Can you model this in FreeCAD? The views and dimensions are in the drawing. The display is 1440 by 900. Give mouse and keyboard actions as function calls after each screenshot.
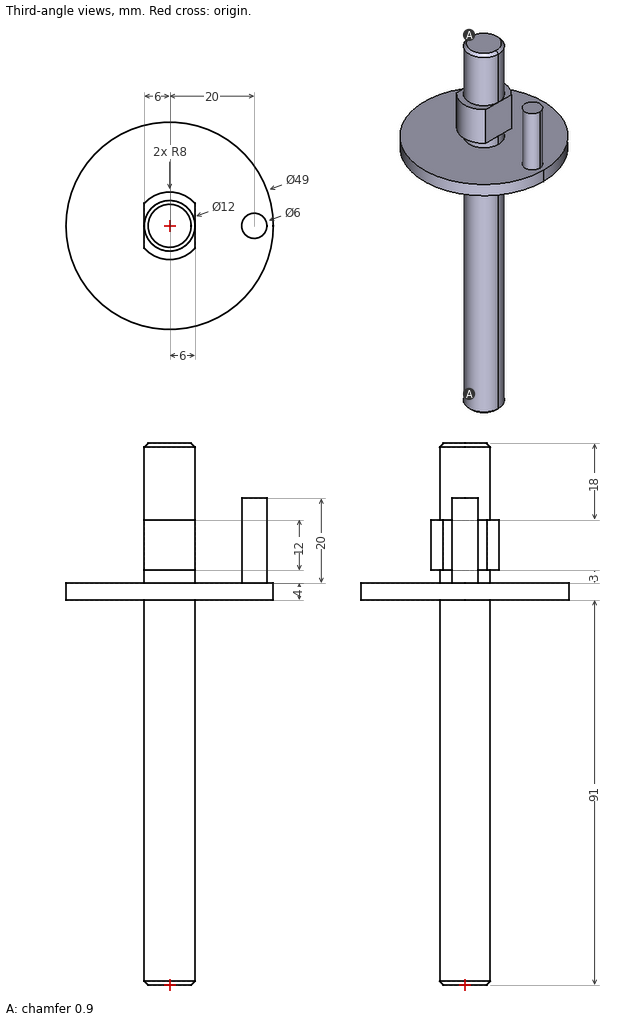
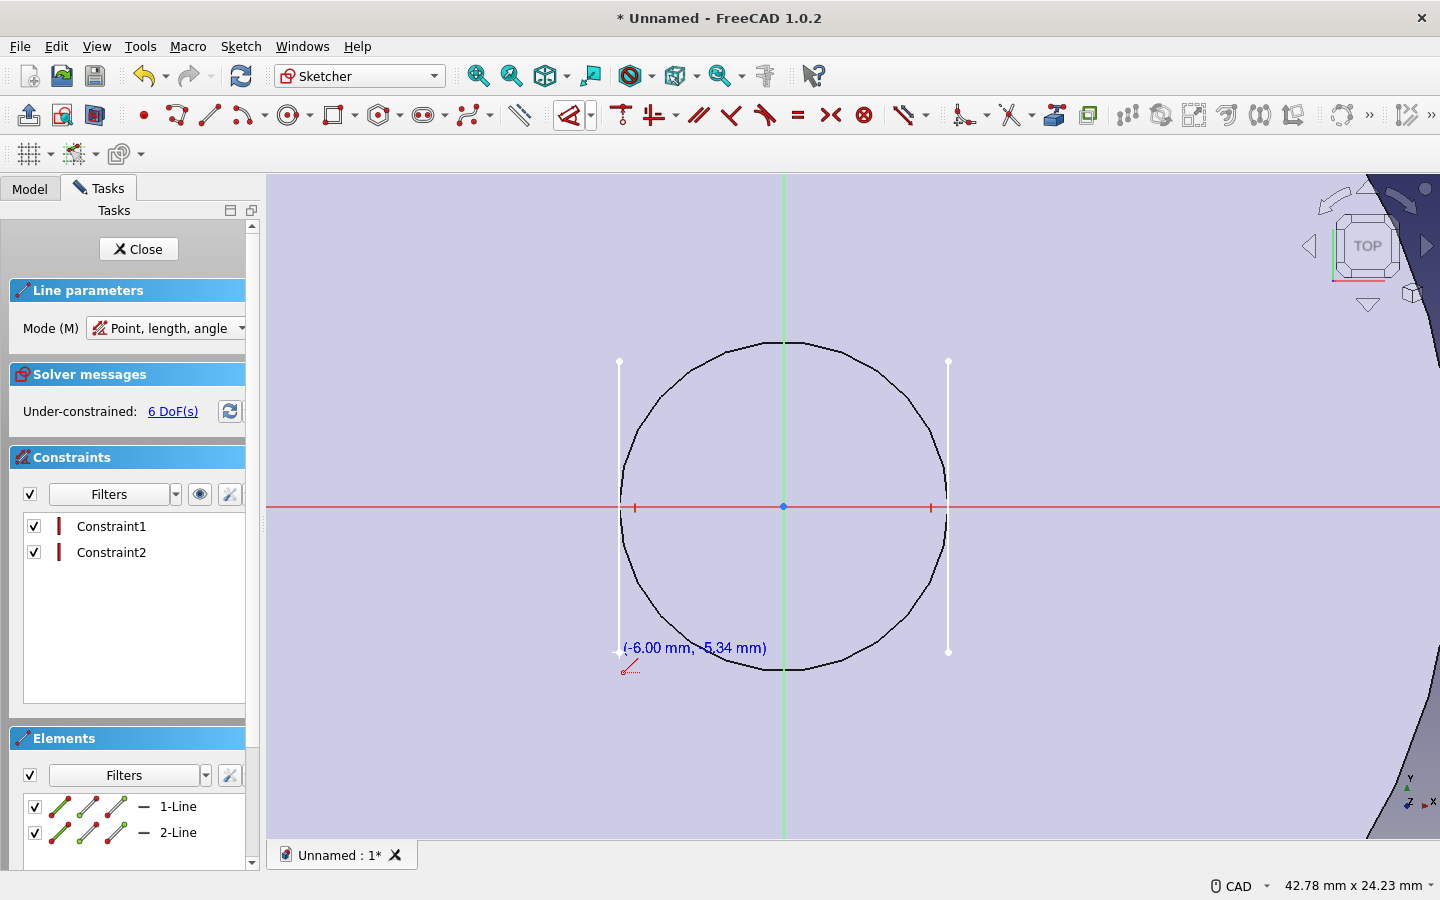
key(g)
key(3)
key(a)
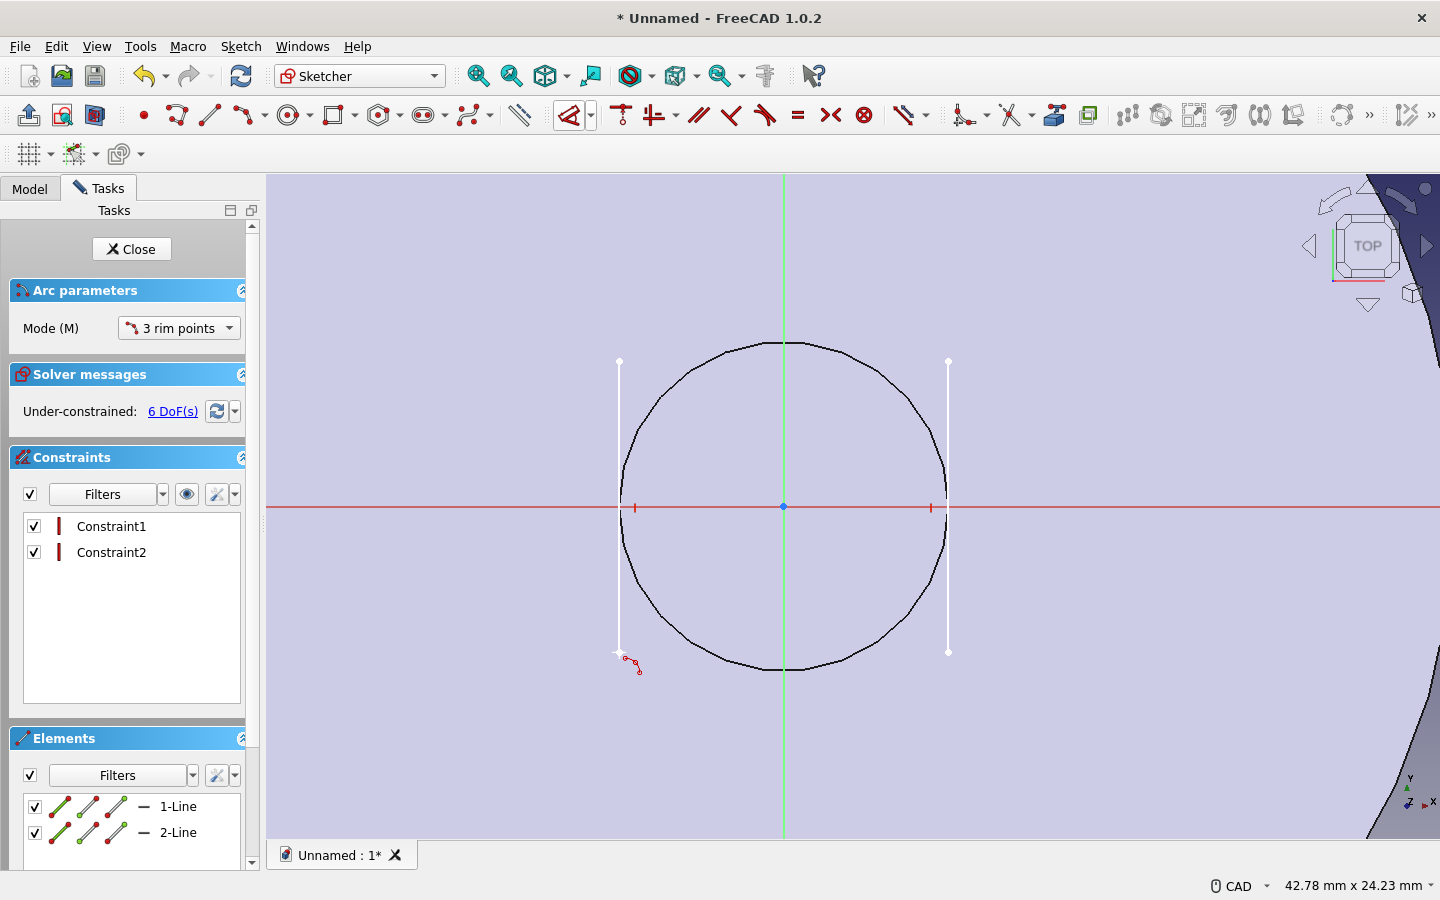
click(948, 362)
click(619, 362)
click(821, 290)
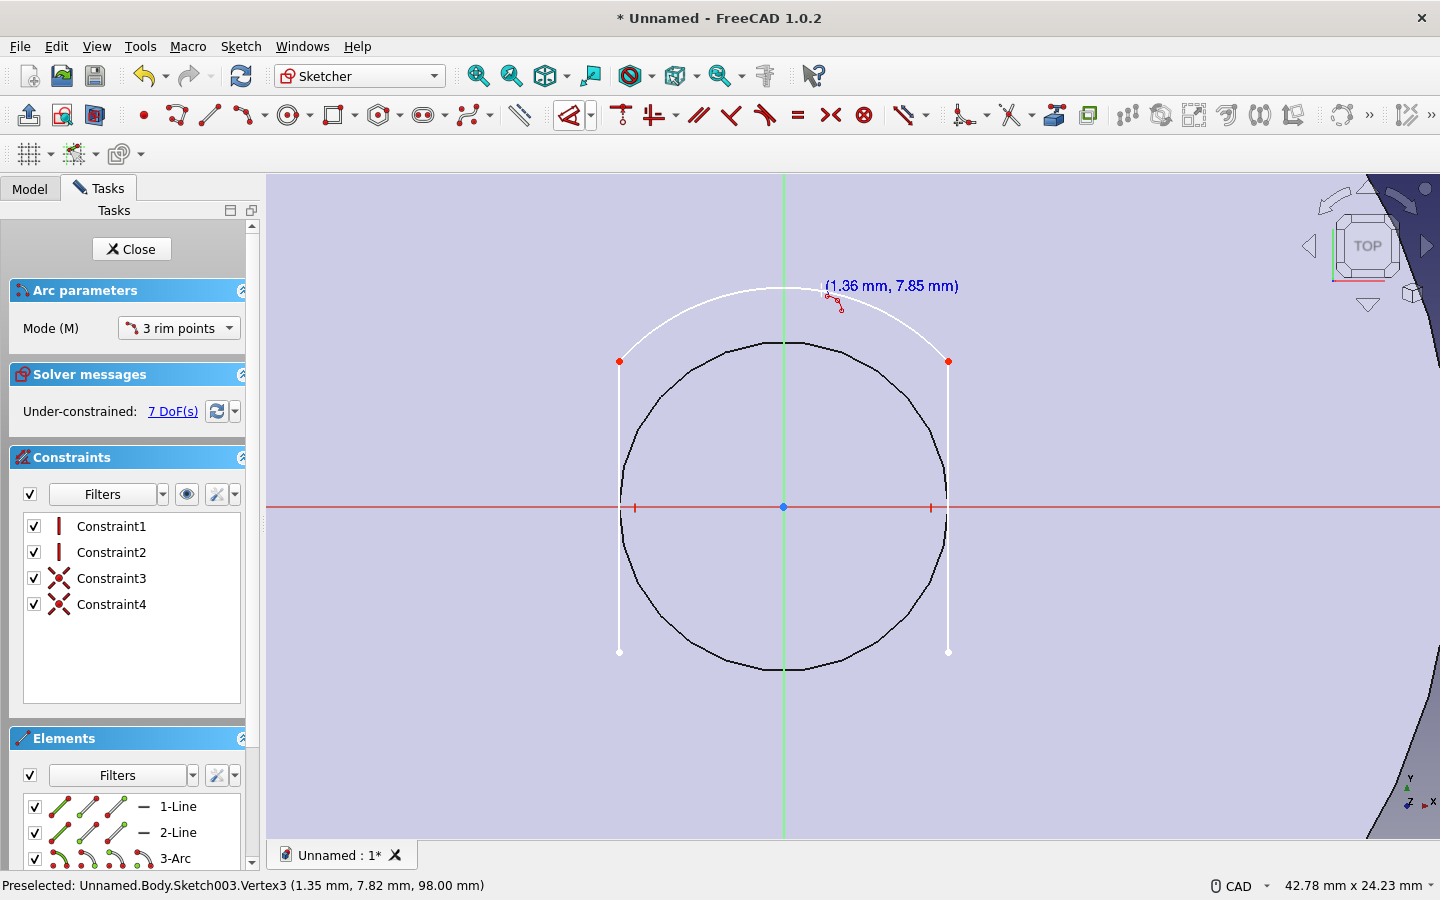
click(619, 653)
click(948, 653)
click(747, 723)
key(Escape)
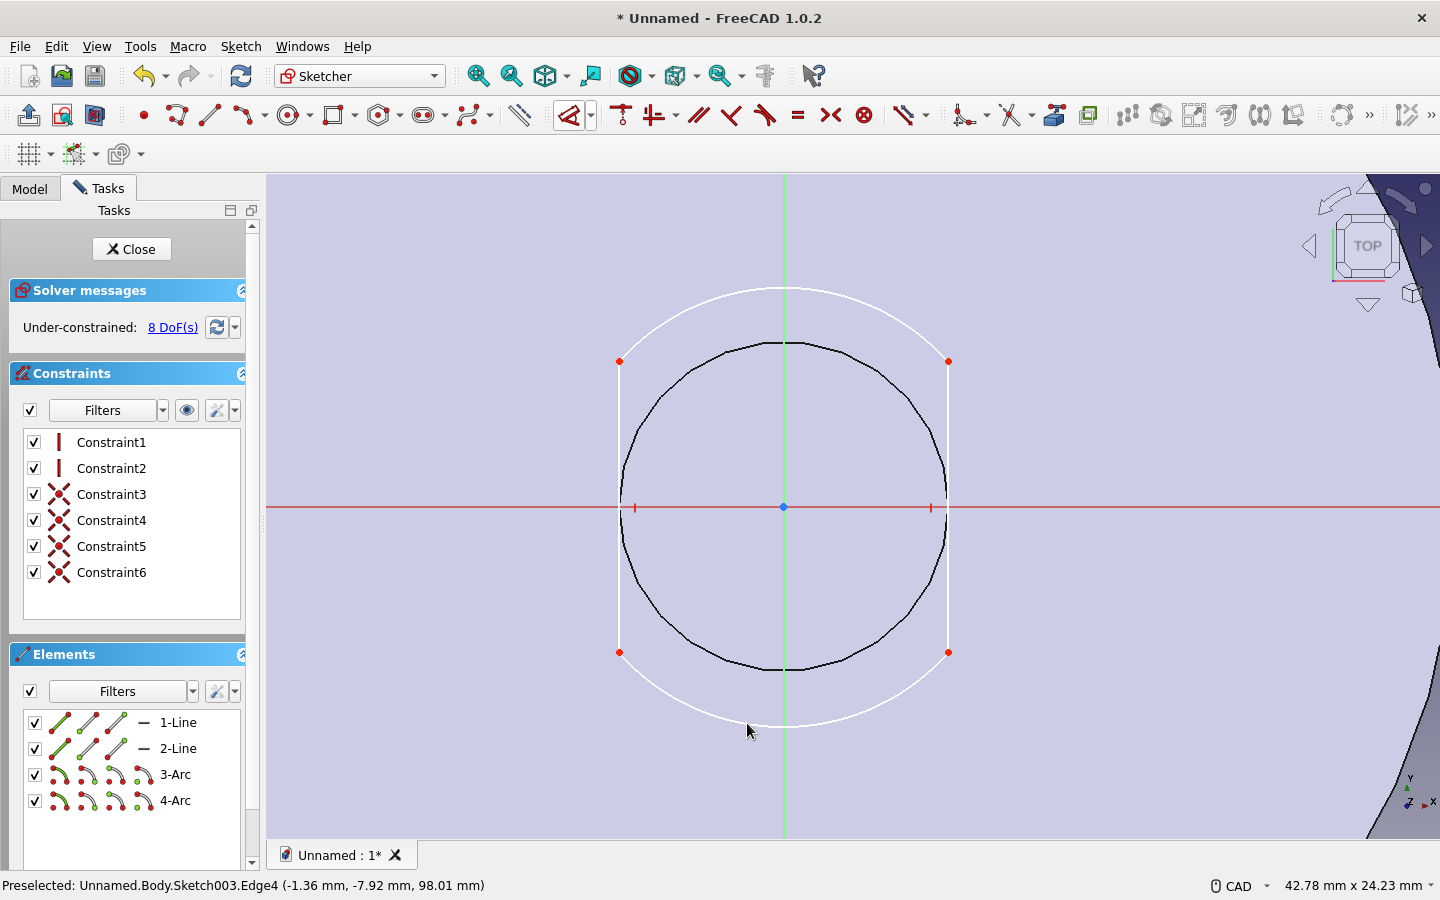
click(856, 300)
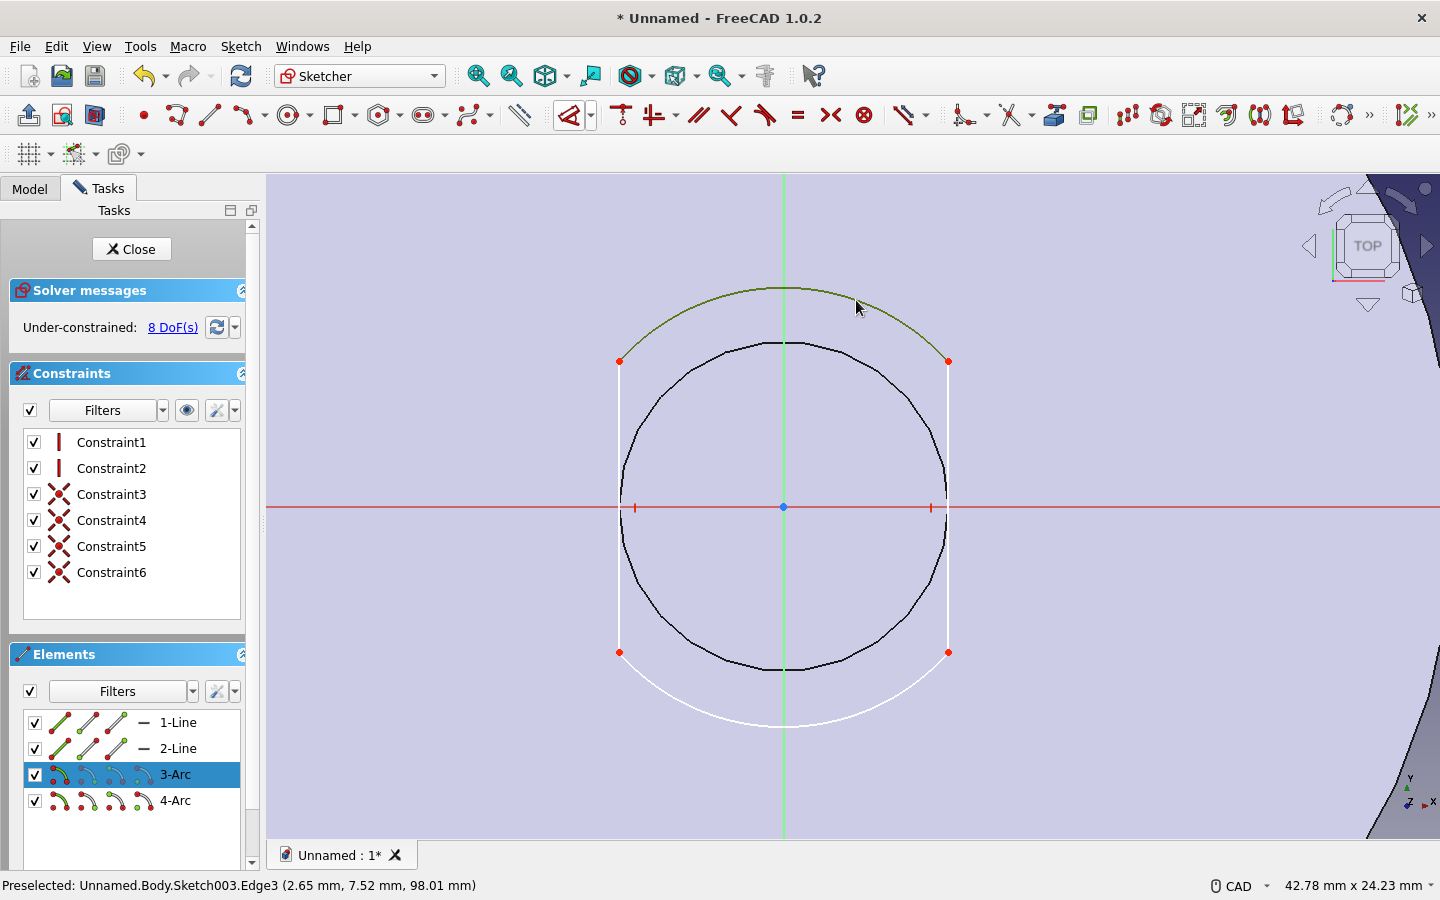
click(711, 715)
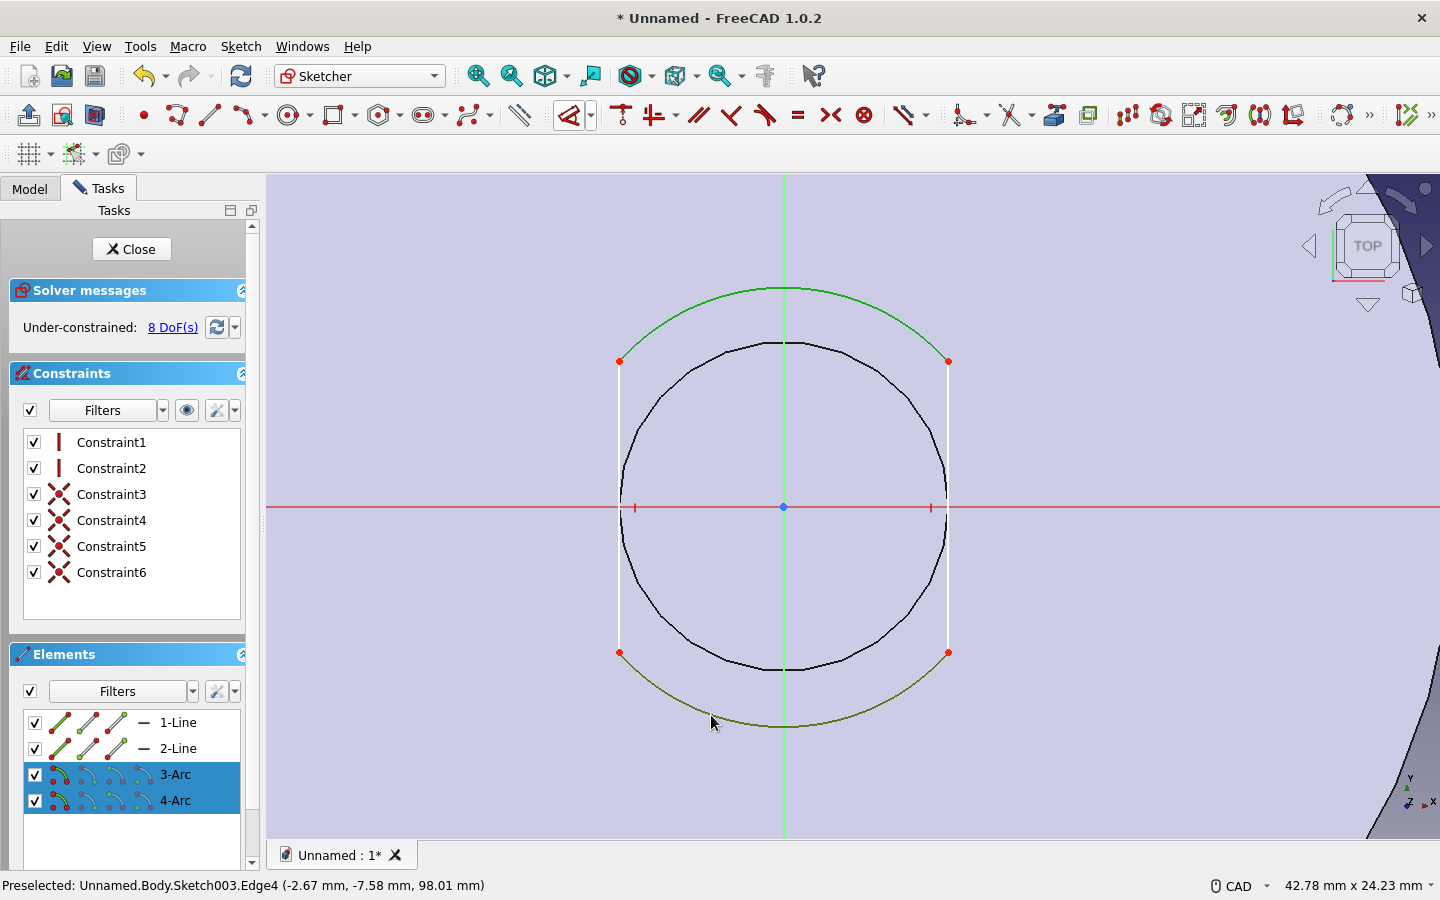
click(621, 116)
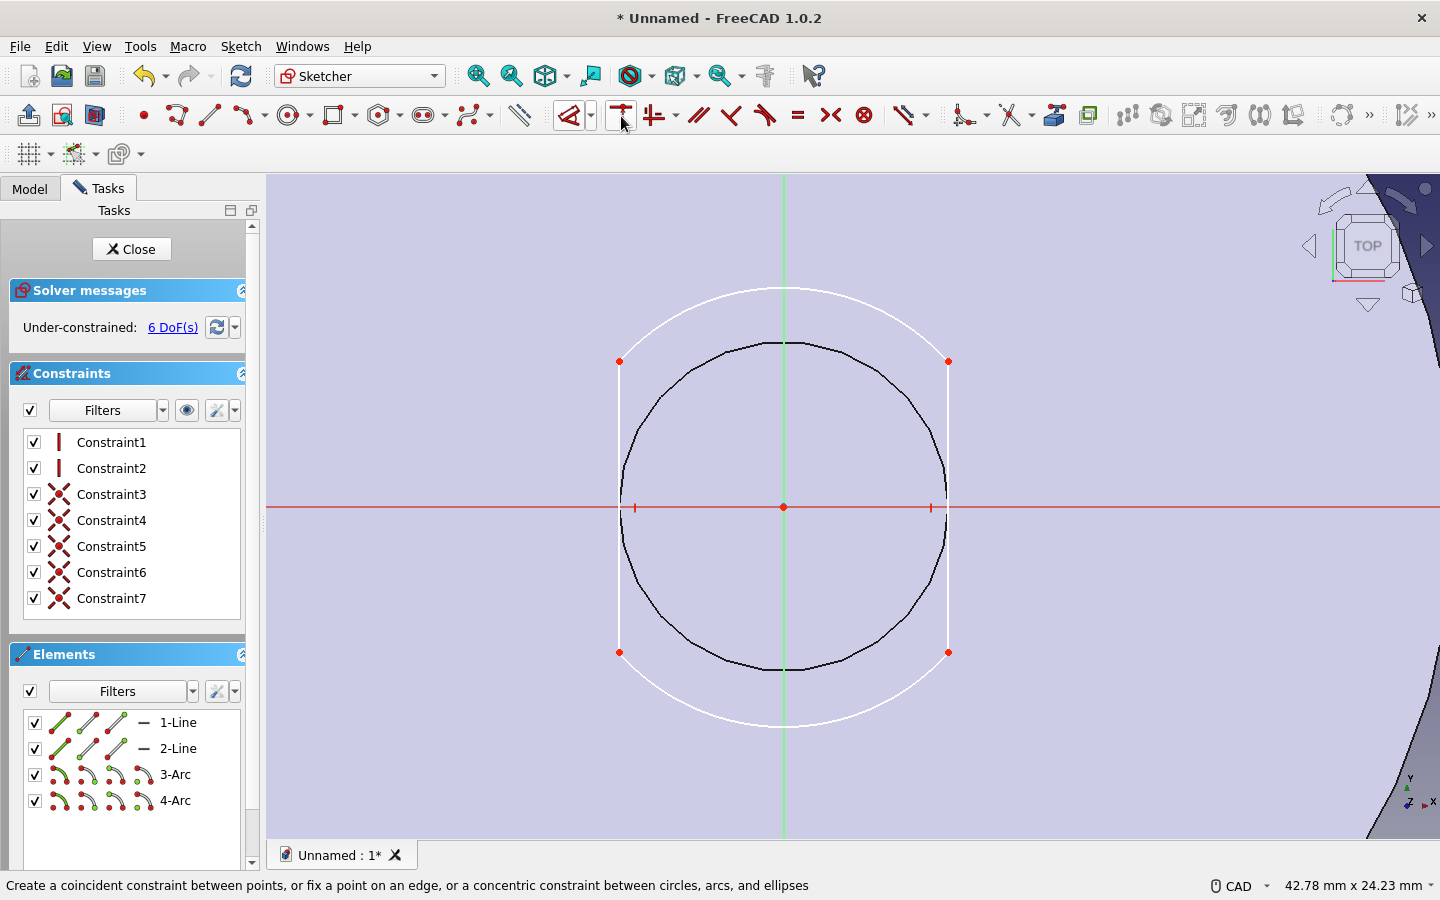
drag(774, 496, 794, 517)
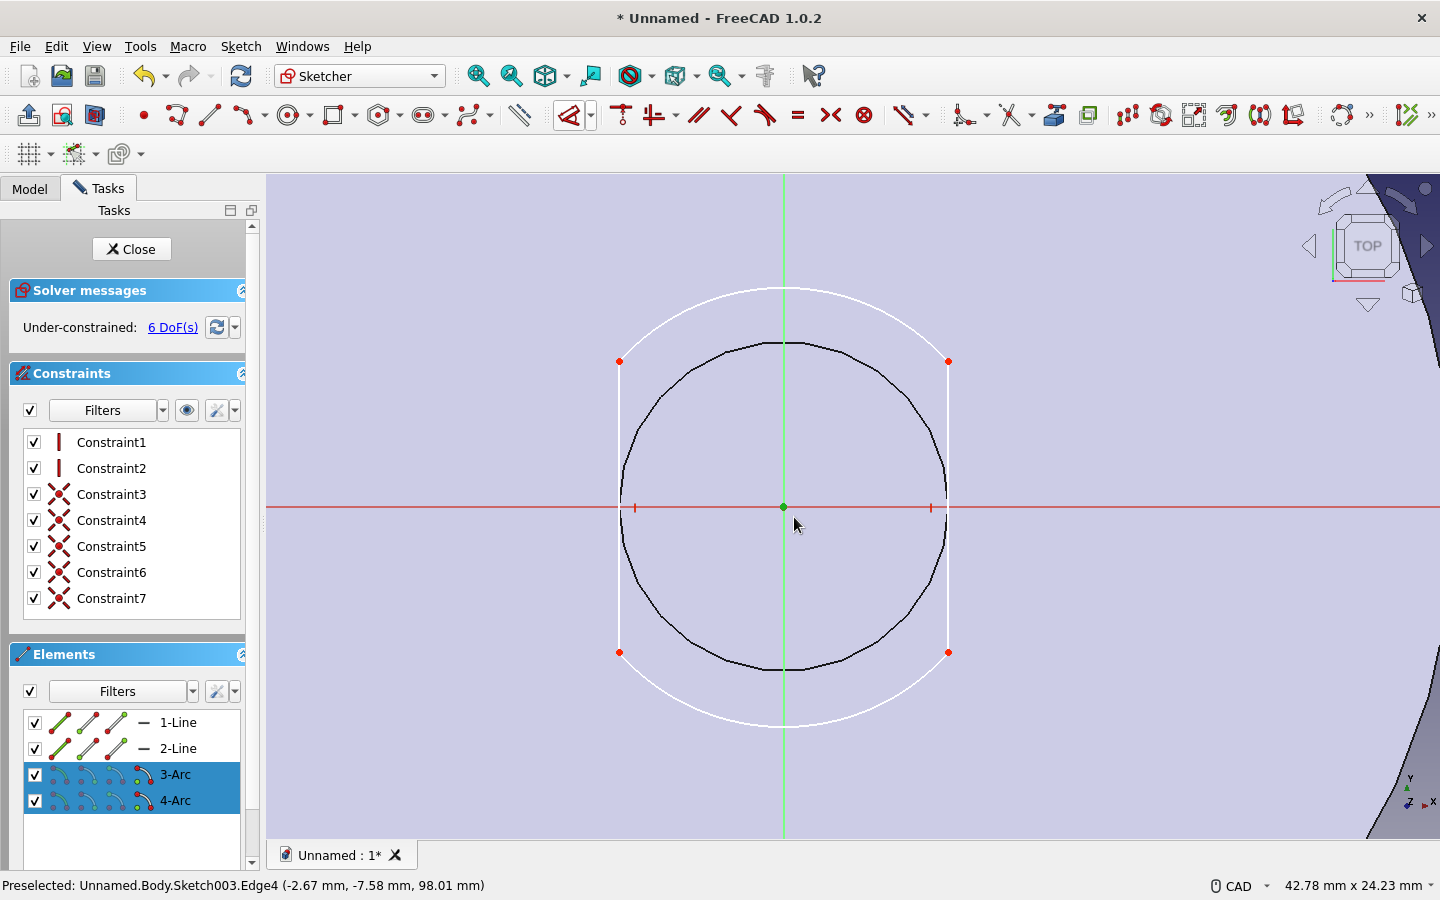
key(c)